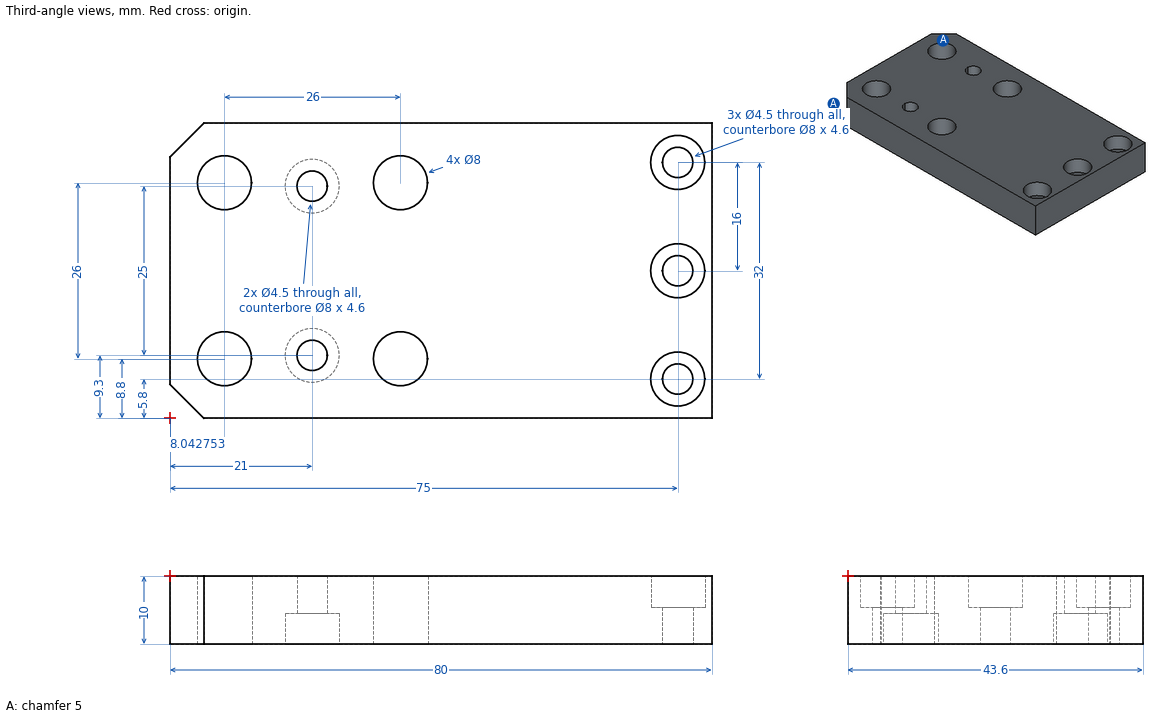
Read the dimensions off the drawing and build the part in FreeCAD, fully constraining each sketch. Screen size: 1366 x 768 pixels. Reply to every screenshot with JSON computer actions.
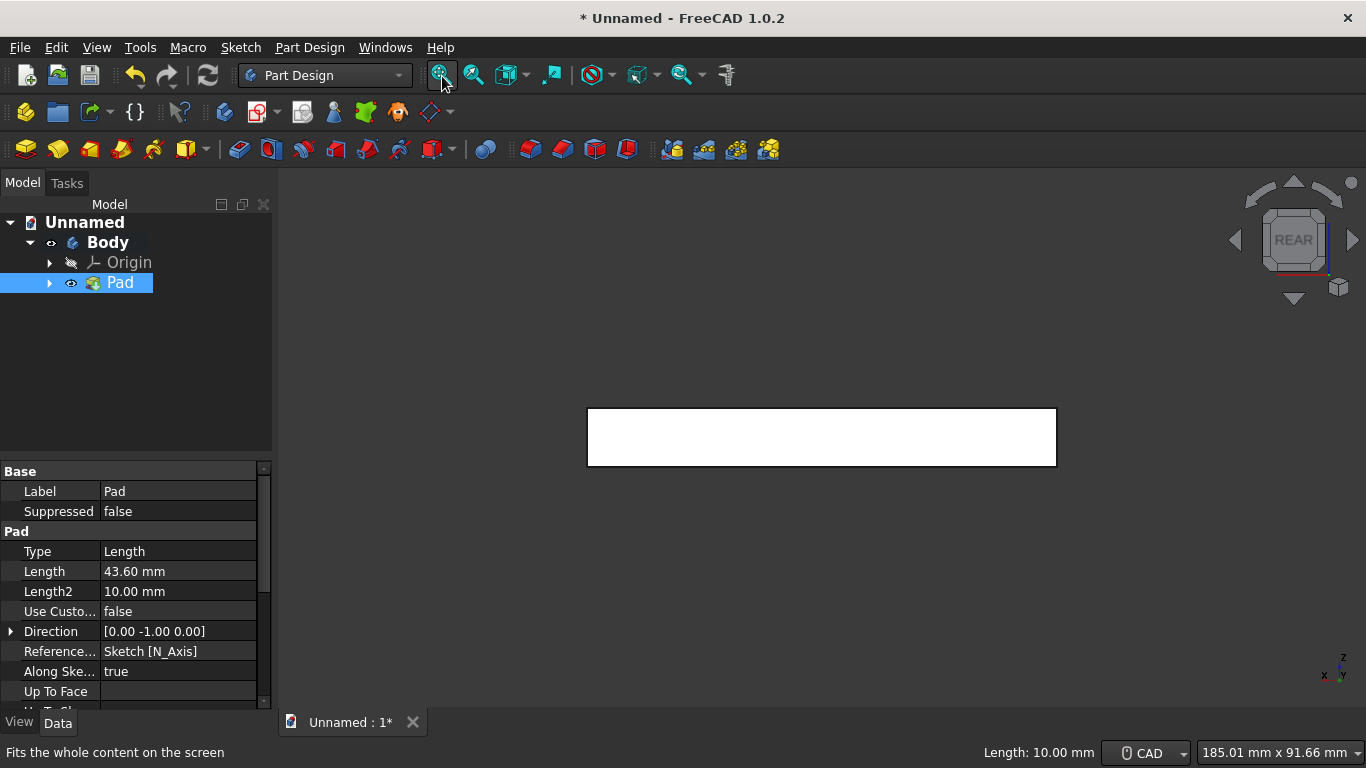
{"action": "left_click", "coordinate": [442, 76]}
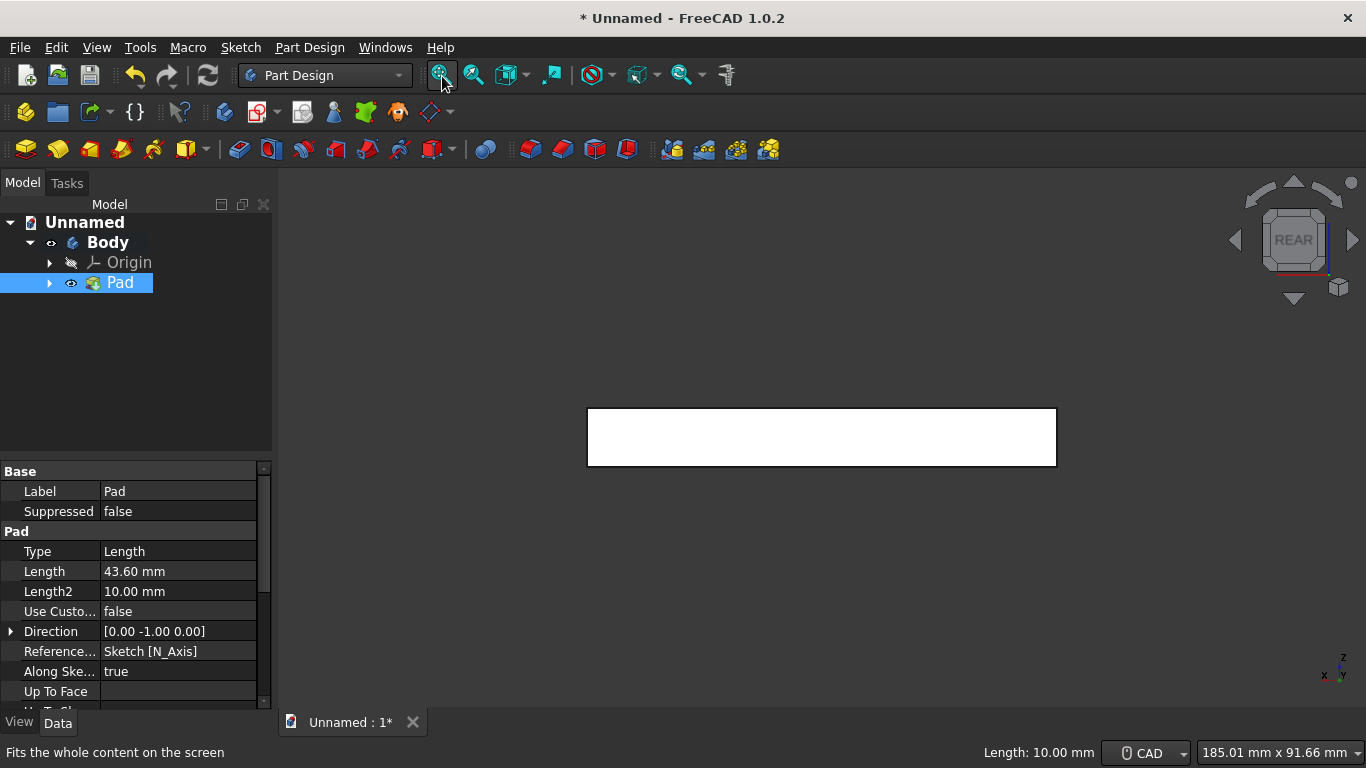
{"action": "left_click", "coordinate": [1057, 437], "text": "ctrl"}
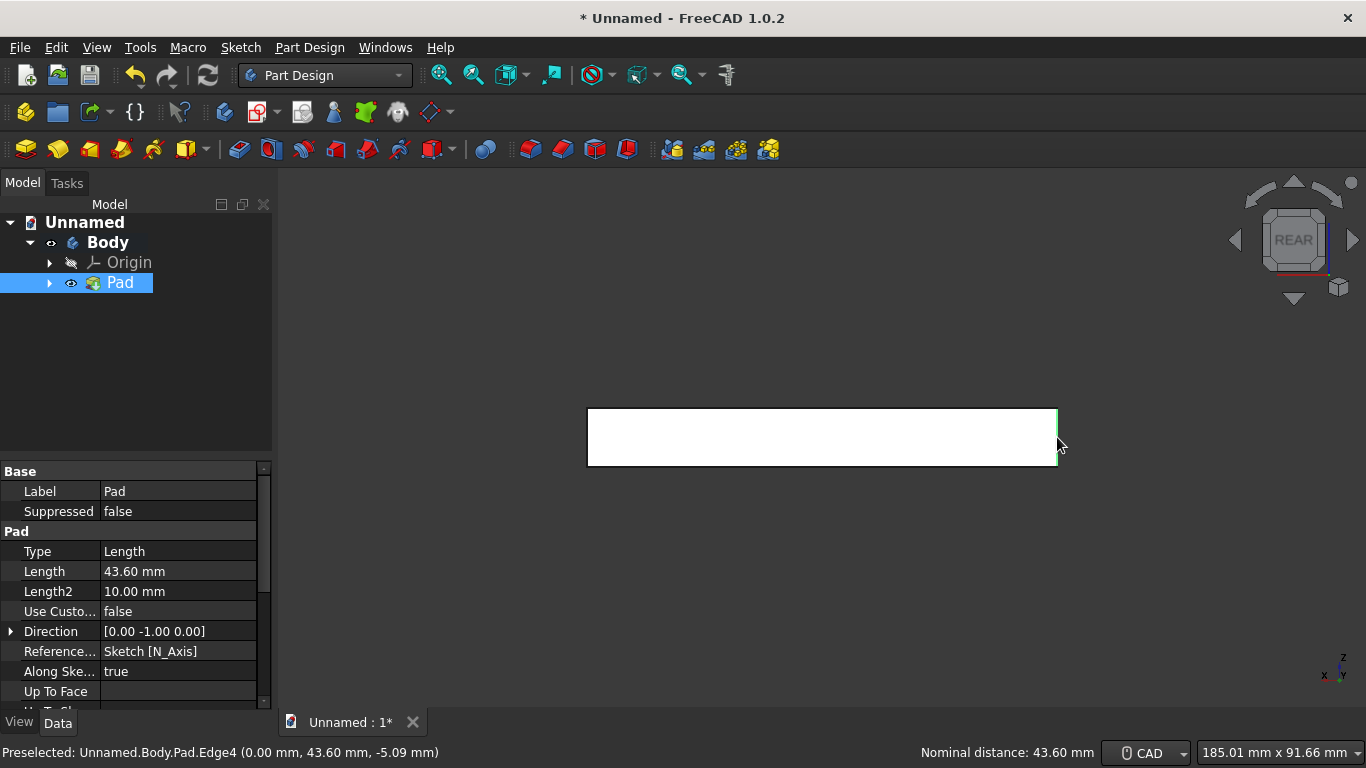
{"action": "left_click", "coordinate": [564, 150]}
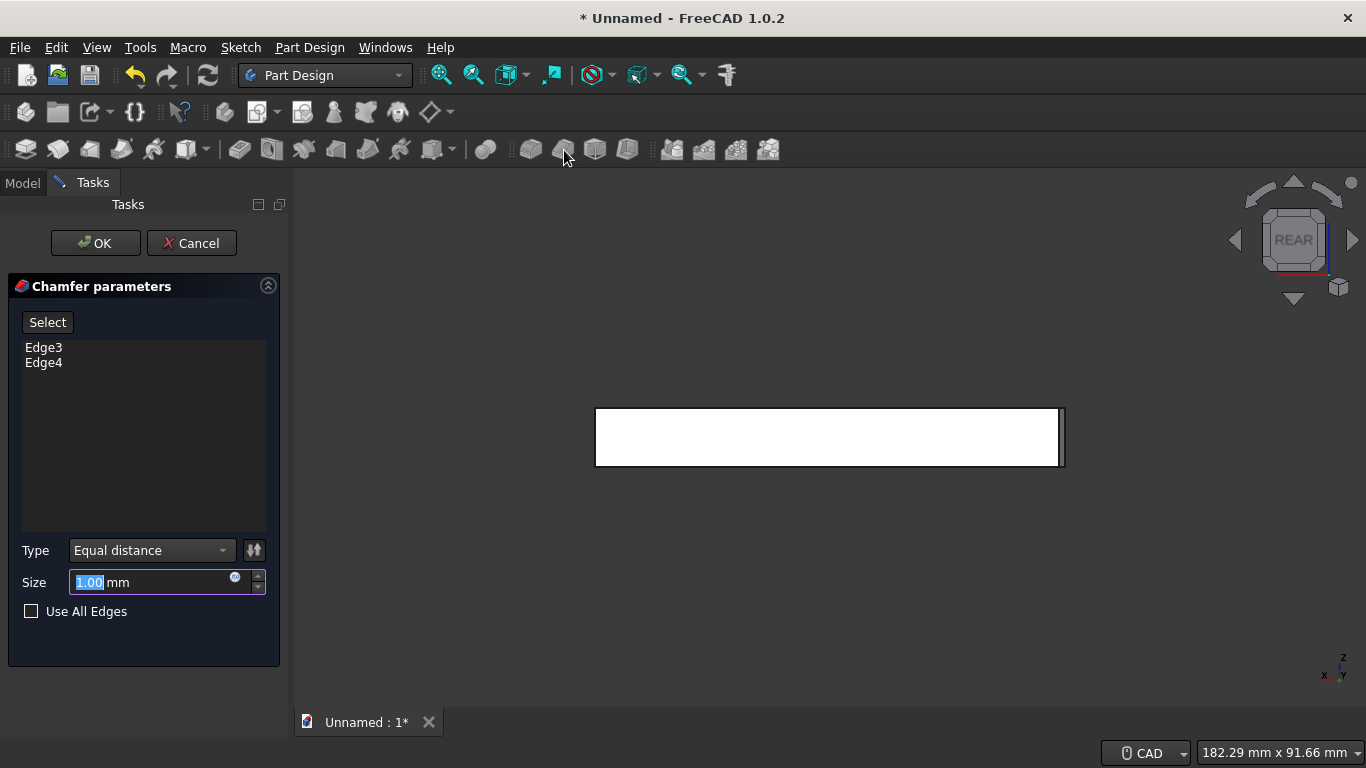
{"action": "type", "text": "5"}
{"action": "key", "text": "Tab"}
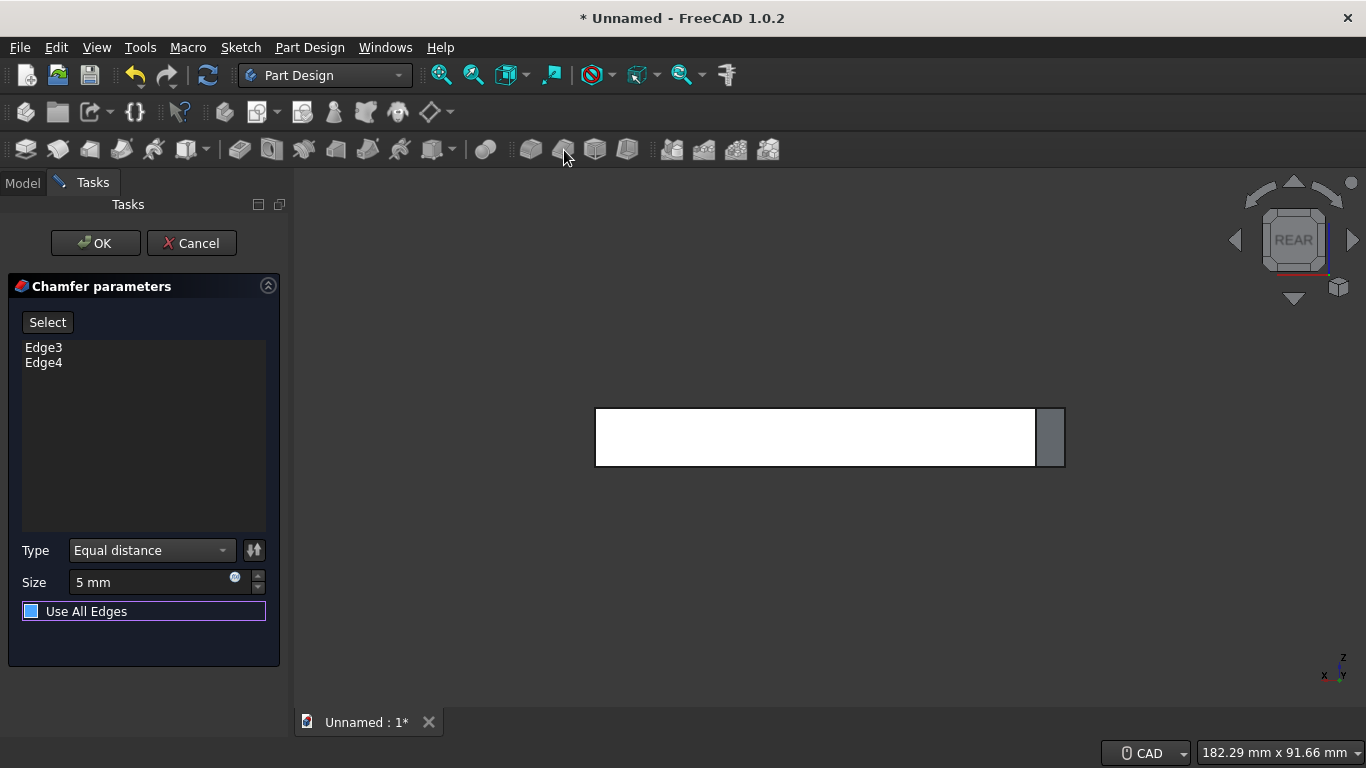
{"action": "left_click", "coordinate": [96, 243]}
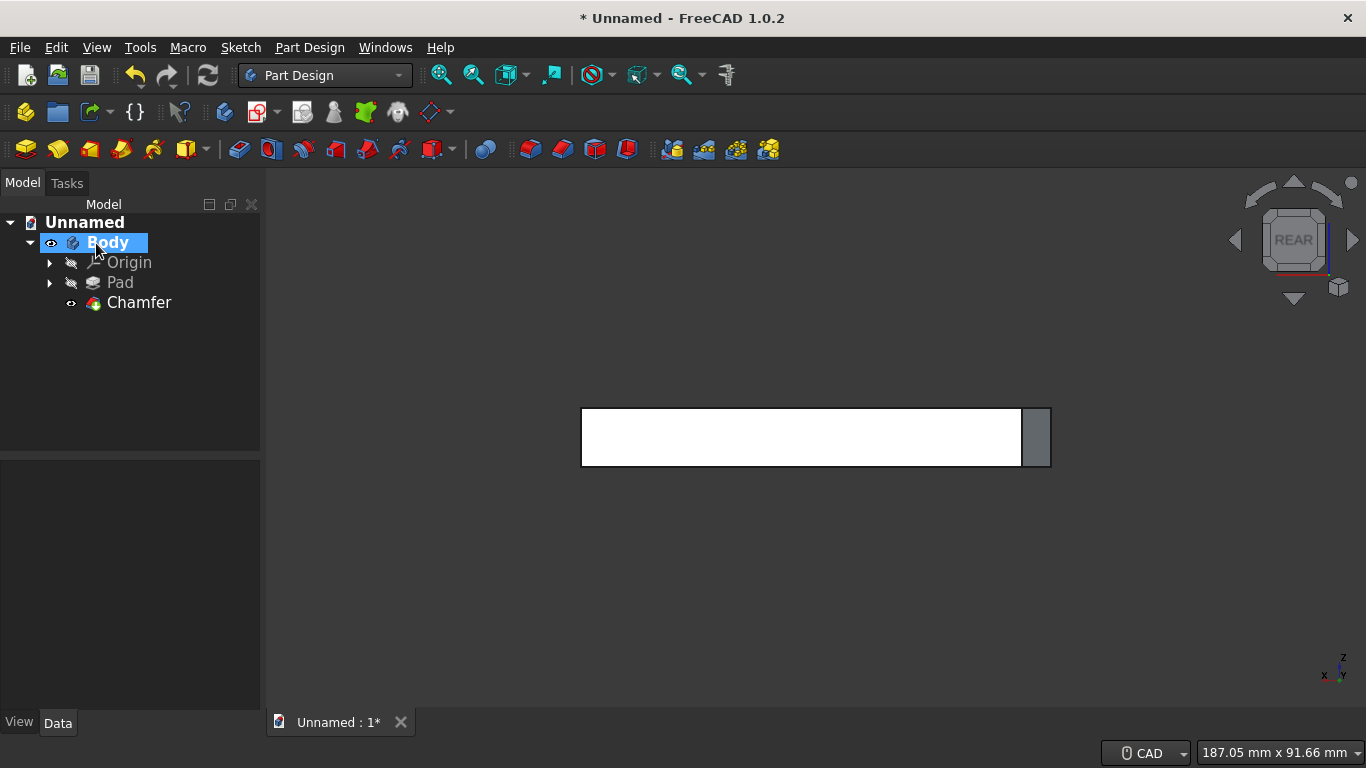
{"action": "left_click", "coordinate": [442, 76]}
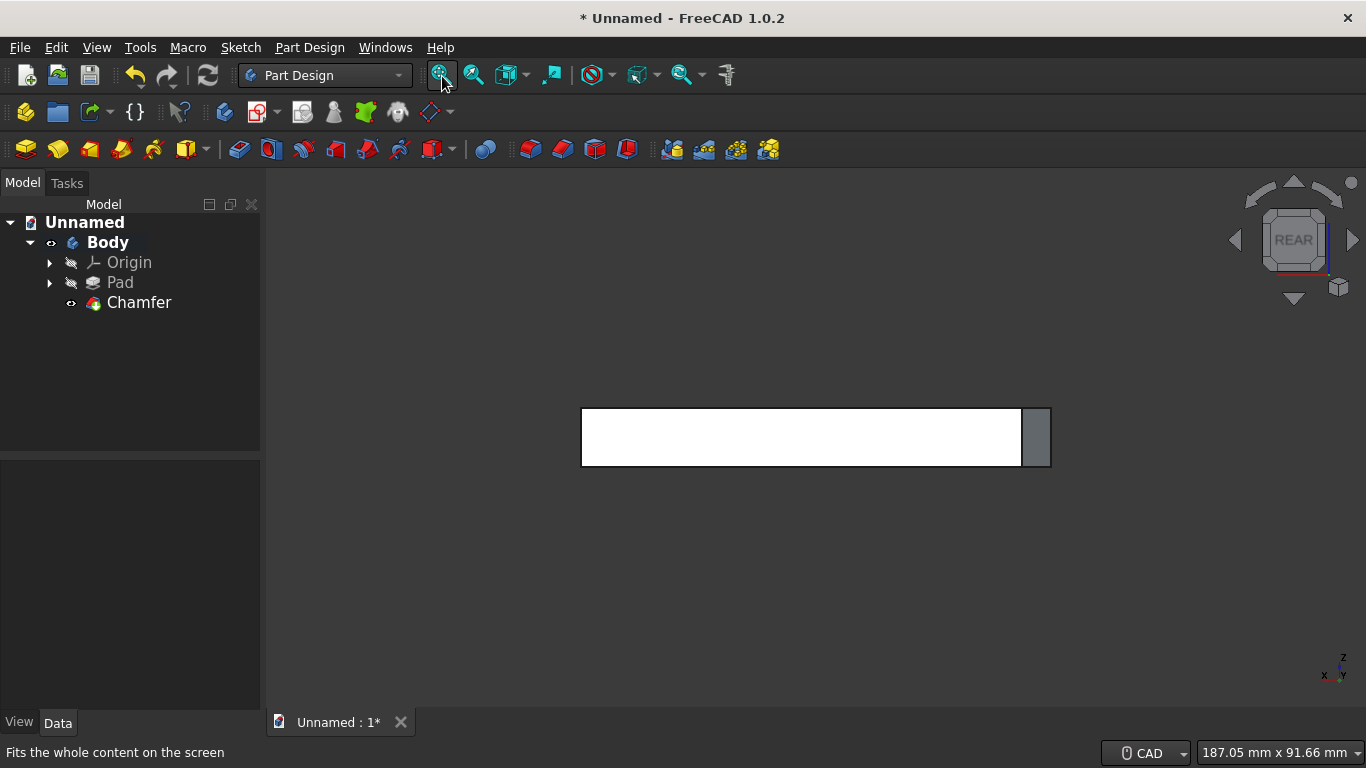
{"action": "key", "text": "5"}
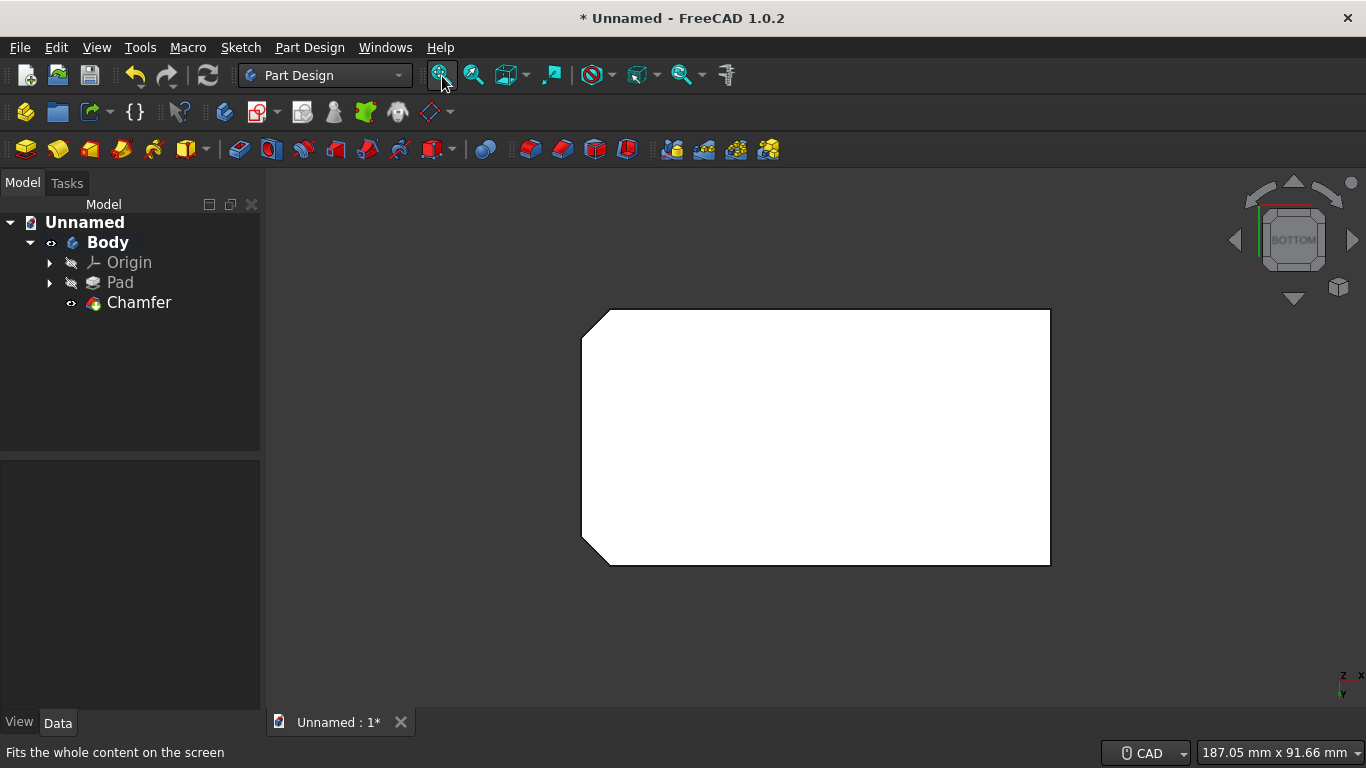
{"action": "left_click", "coordinate": [883, 436]}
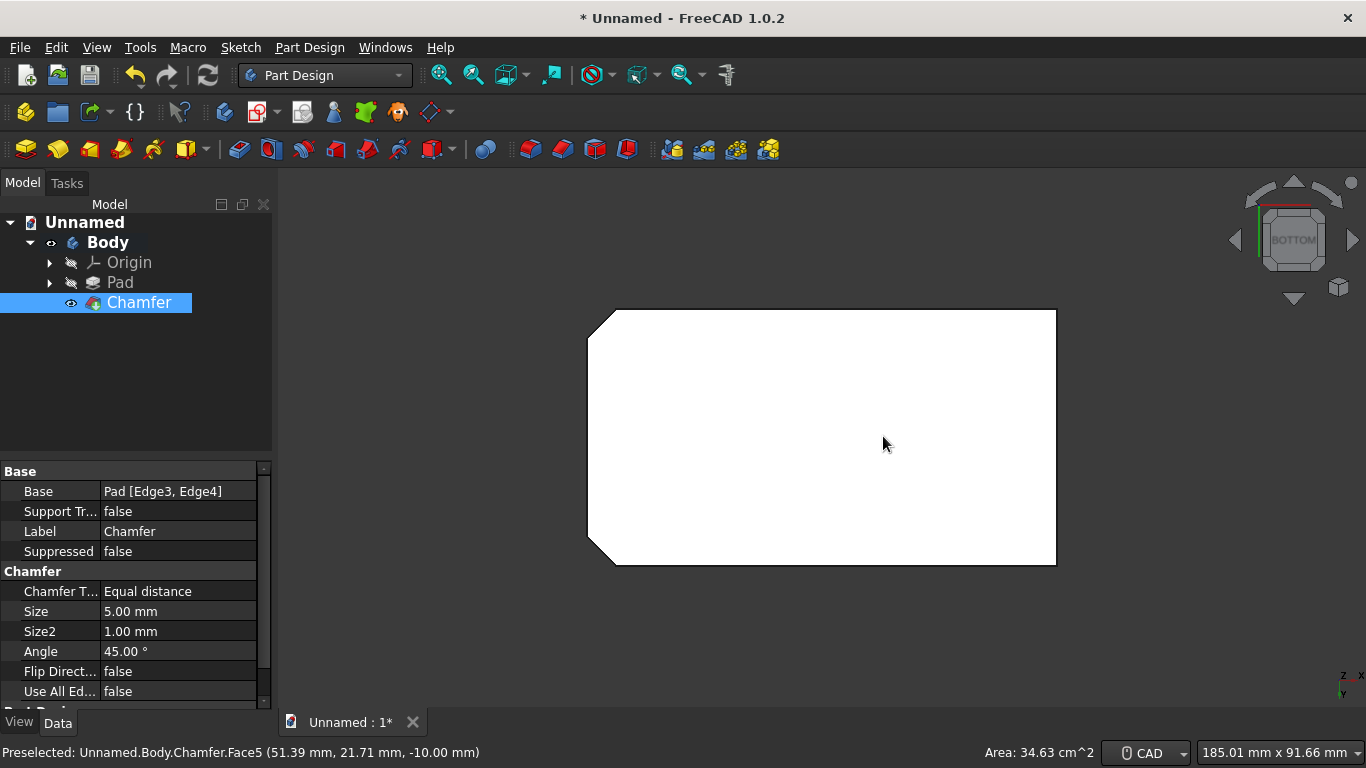
{"action": "left_click", "coordinate": [258, 112]}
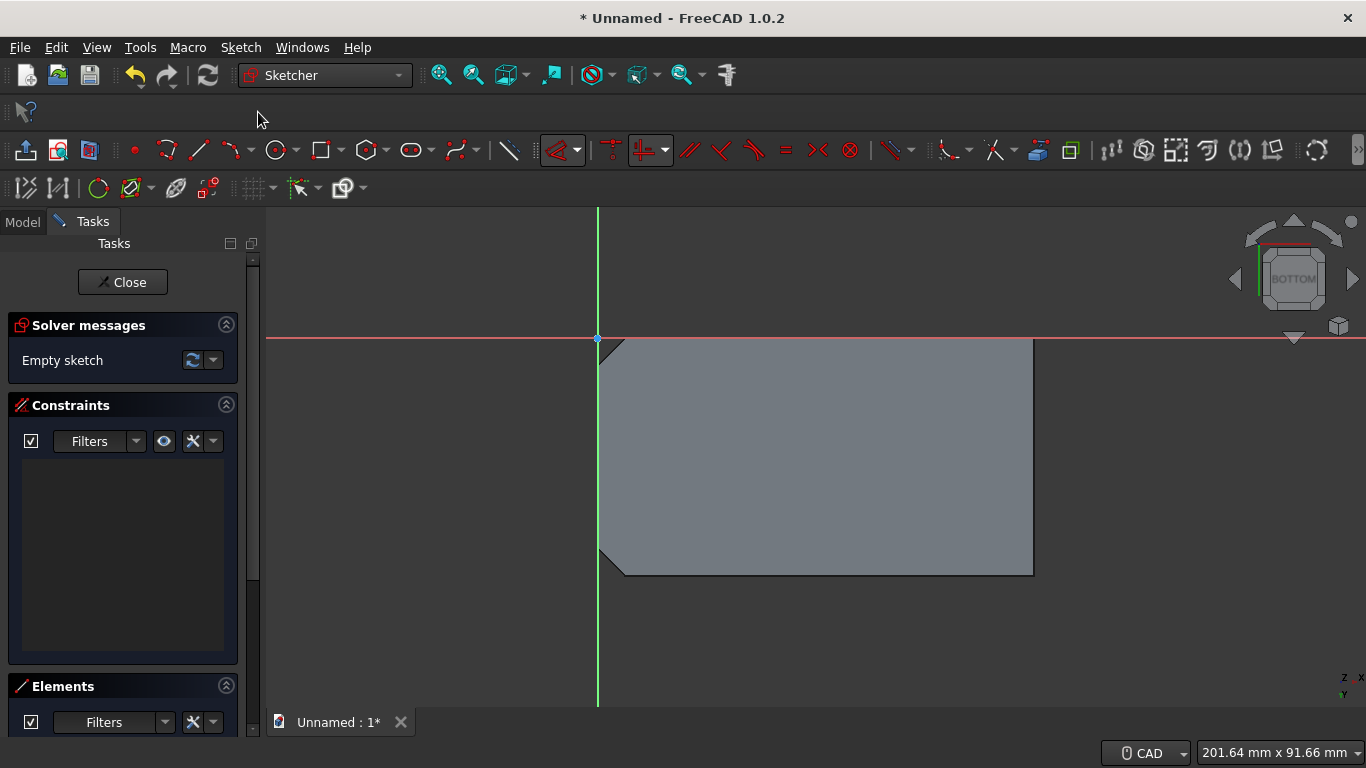
{"action": "scroll", "coordinate": [608, 417], "scroll_direction": "up", "scroll_amount": 2}